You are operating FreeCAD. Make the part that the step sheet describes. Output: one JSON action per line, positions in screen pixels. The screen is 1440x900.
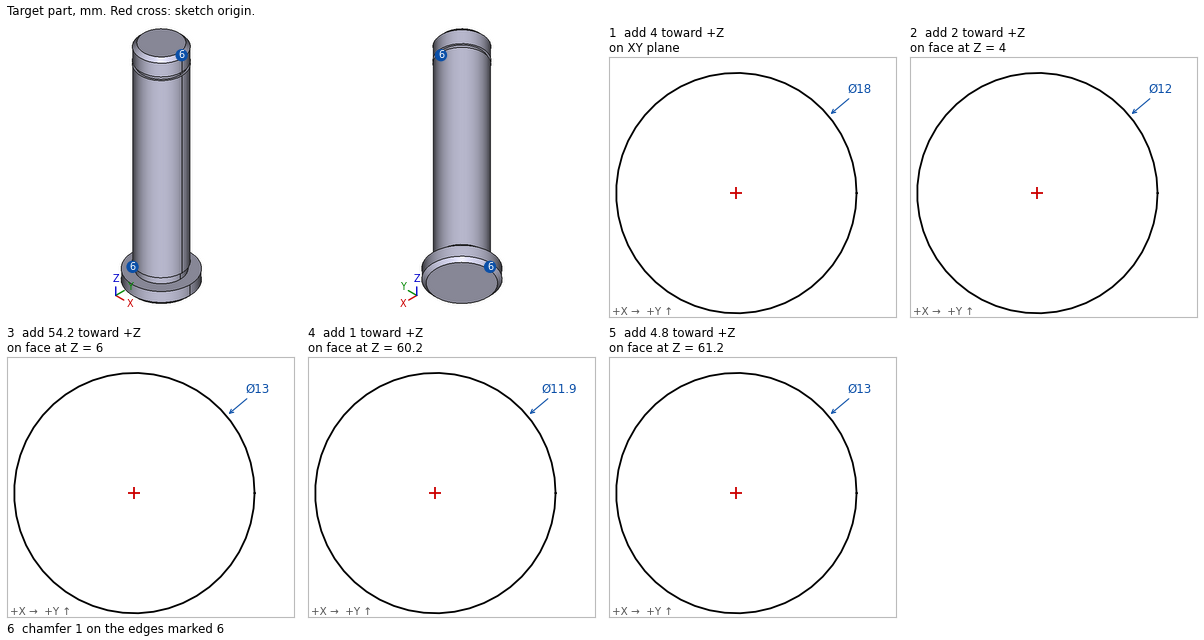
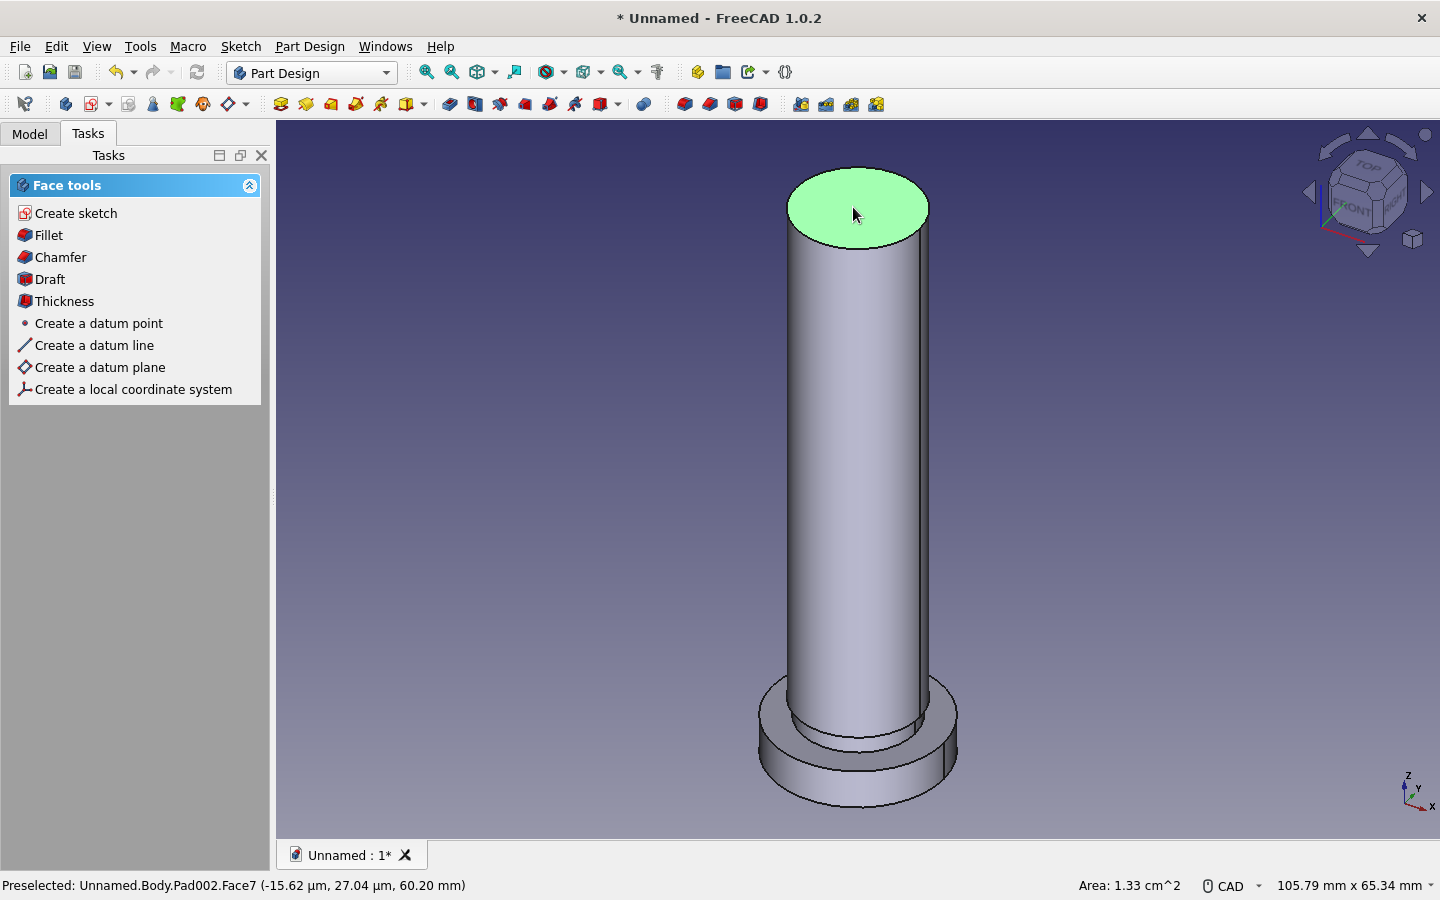
{"action": "left_click", "coordinate": [90, 104]}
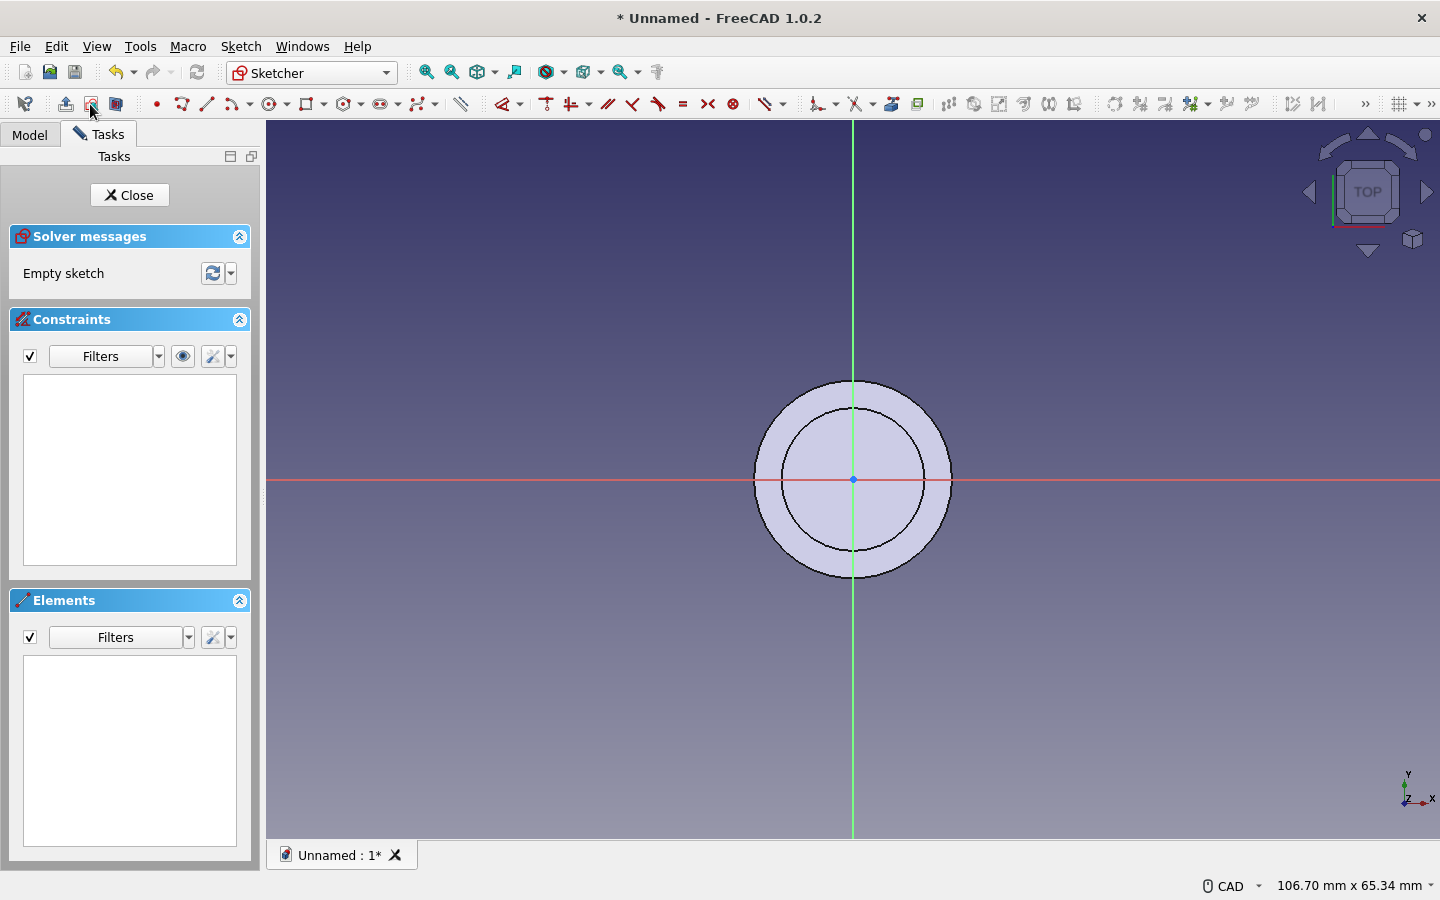
{"action": "scroll", "coordinate": [883, 480], "scroll_direction": "up", "scroll_amount": 6}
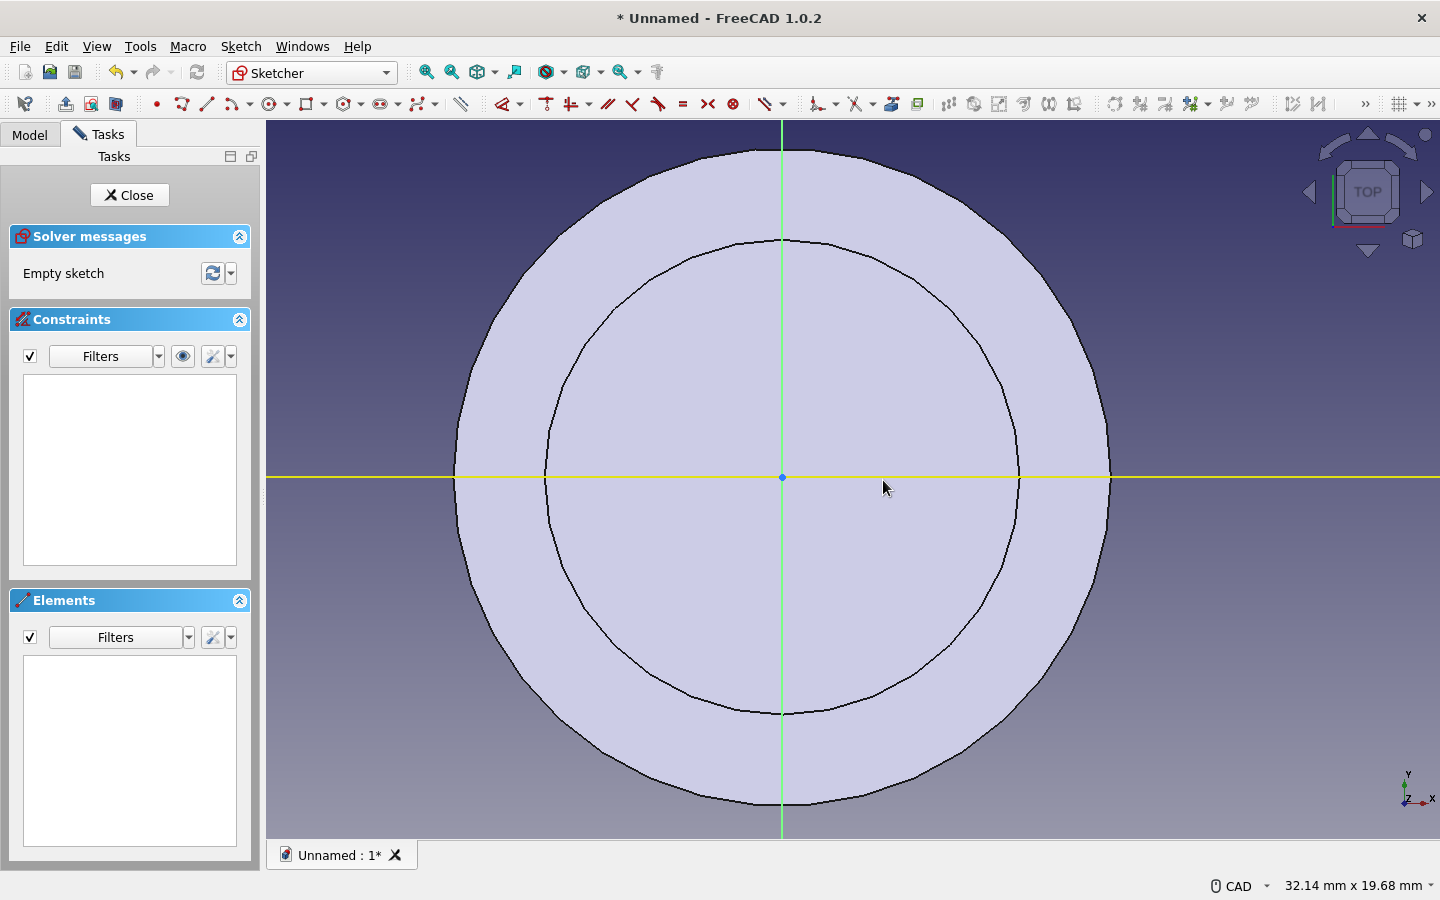
{"action": "left_click", "coordinate": [268, 104]}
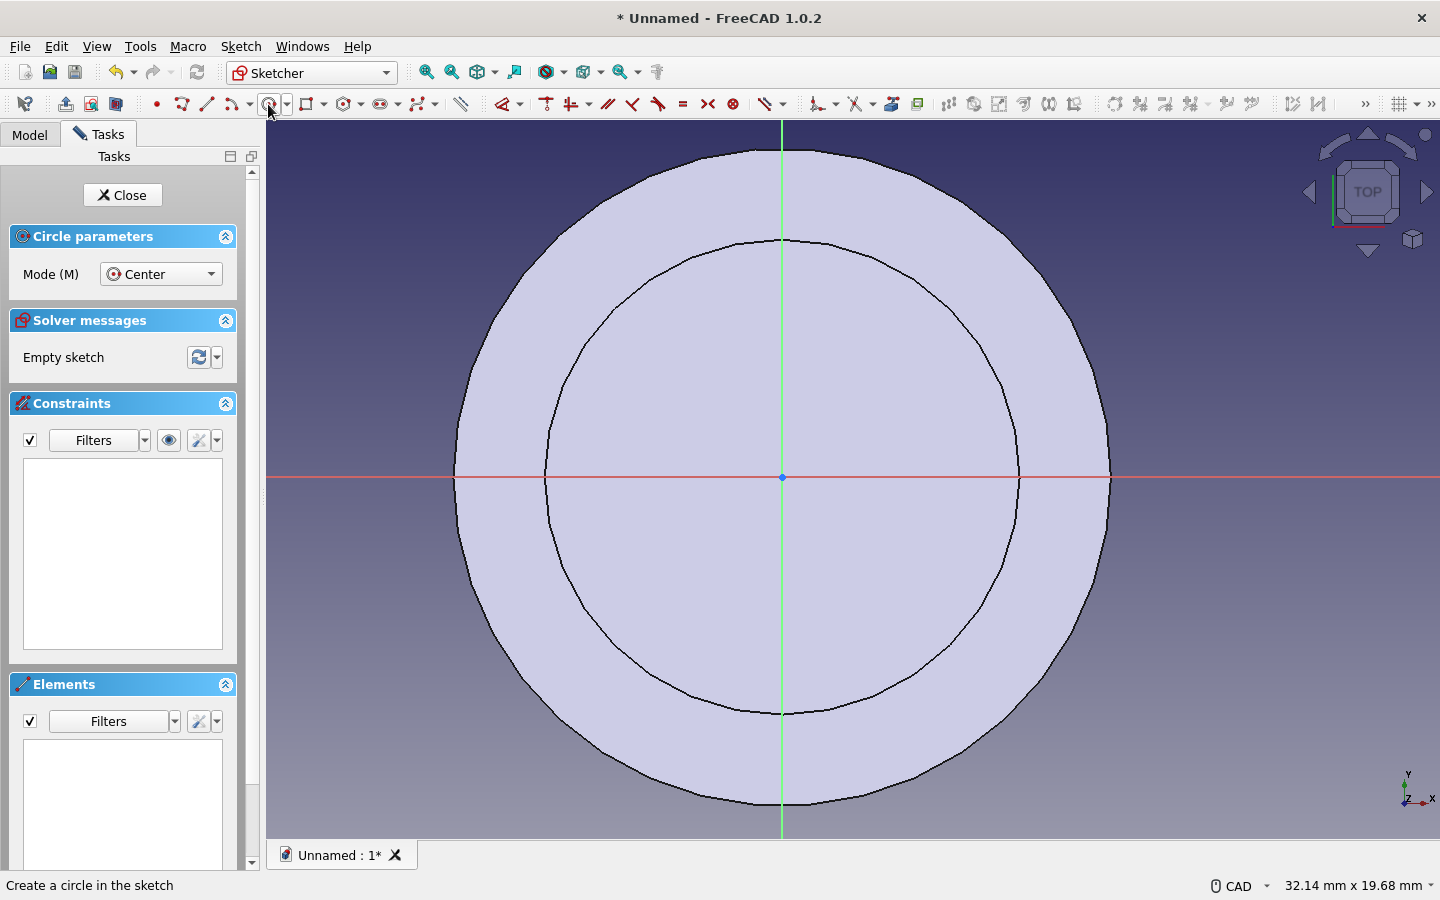
{"action": "left_click", "coordinate": [782, 477]}
{"action": "left_click", "coordinate": [936, 323]}
{"action": "key", "text": "Escape"}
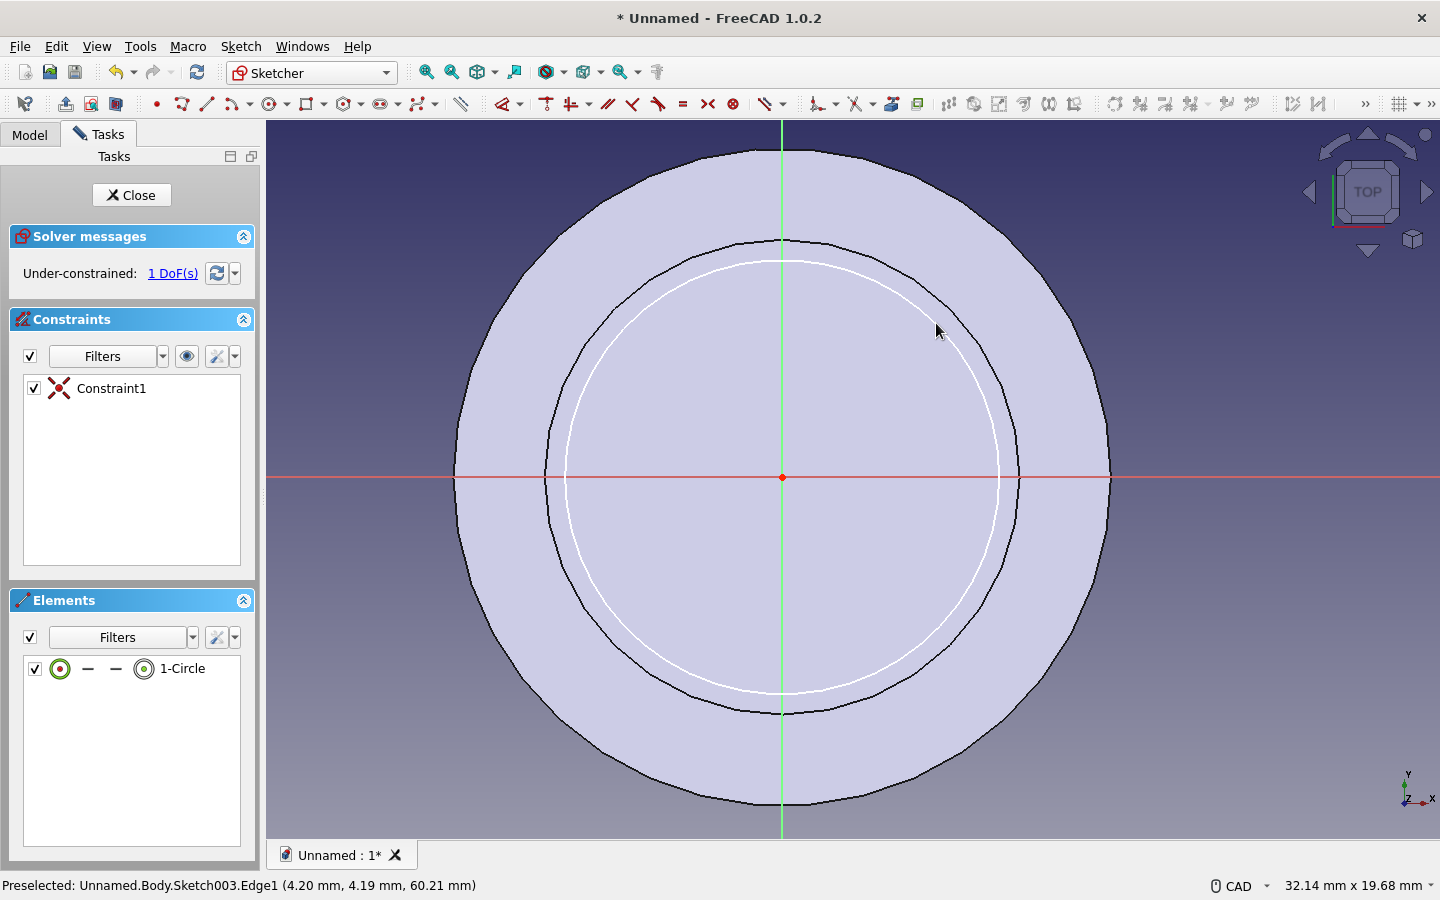
{"action": "left_click", "coordinate": [502, 104]}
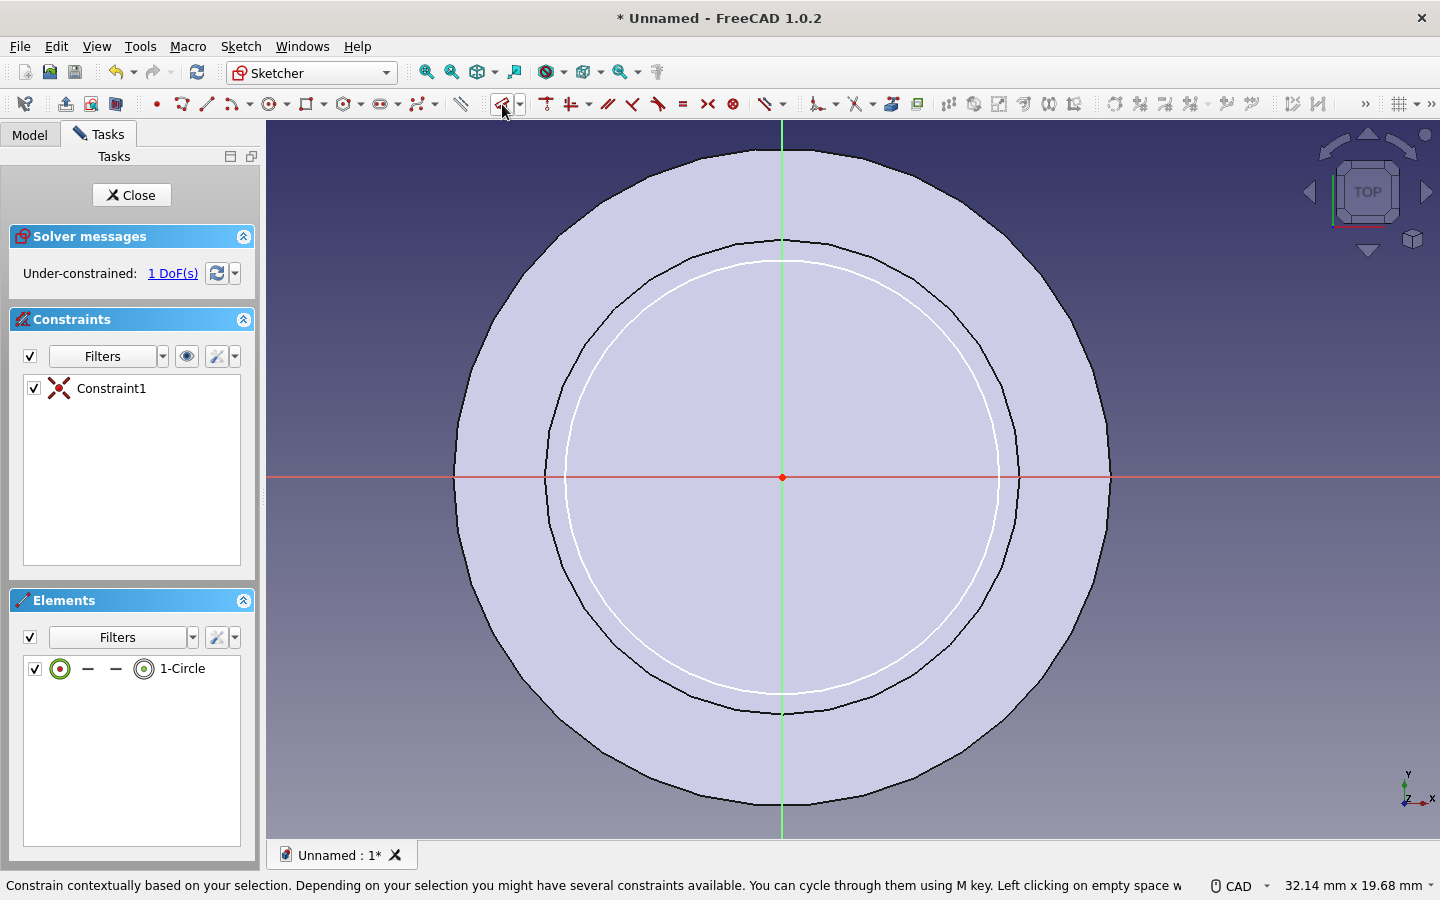
{"action": "left_click", "coordinate": [935, 323]}
{"action": "left_click", "coordinate": [958, 300]}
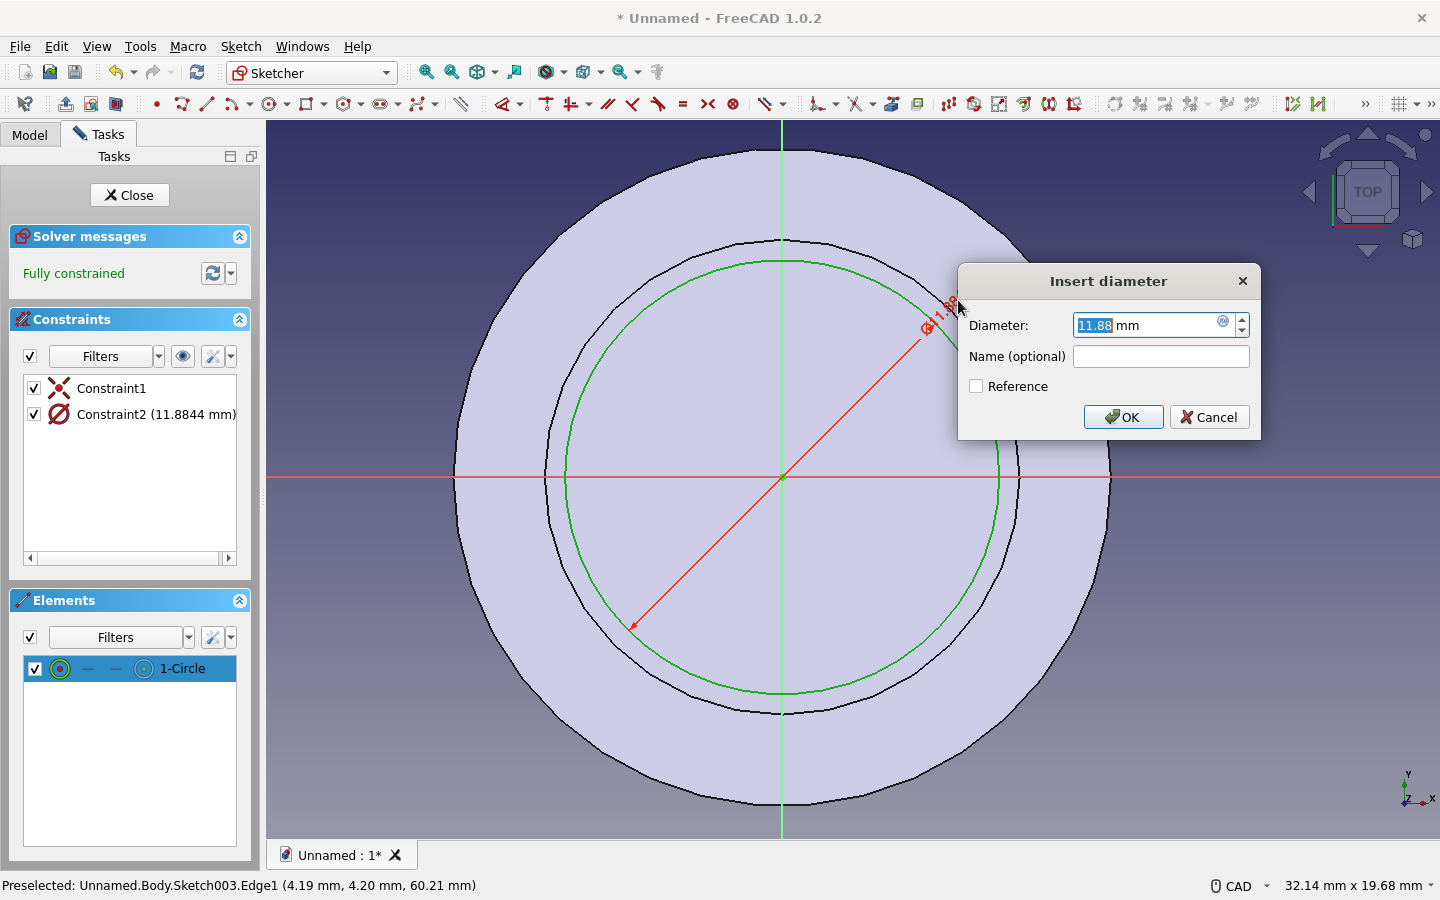
{"action": "type", "text": "11.9"}
{"action": "key", "text": "Return"}
{"action": "key", "text": "Escape"}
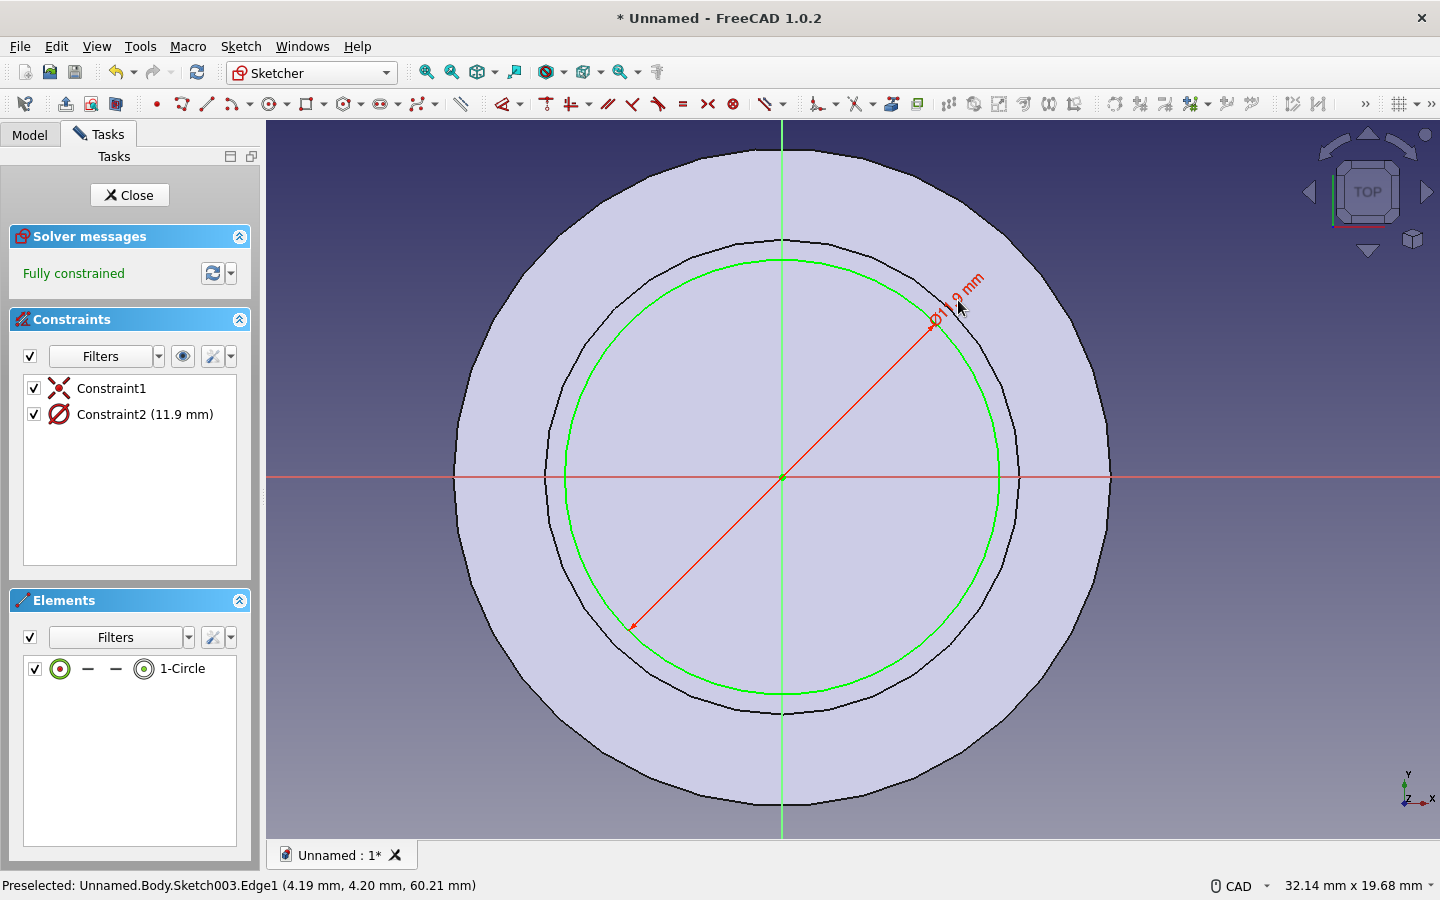
{"action": "left_click", "coordinate": [130, 195]}